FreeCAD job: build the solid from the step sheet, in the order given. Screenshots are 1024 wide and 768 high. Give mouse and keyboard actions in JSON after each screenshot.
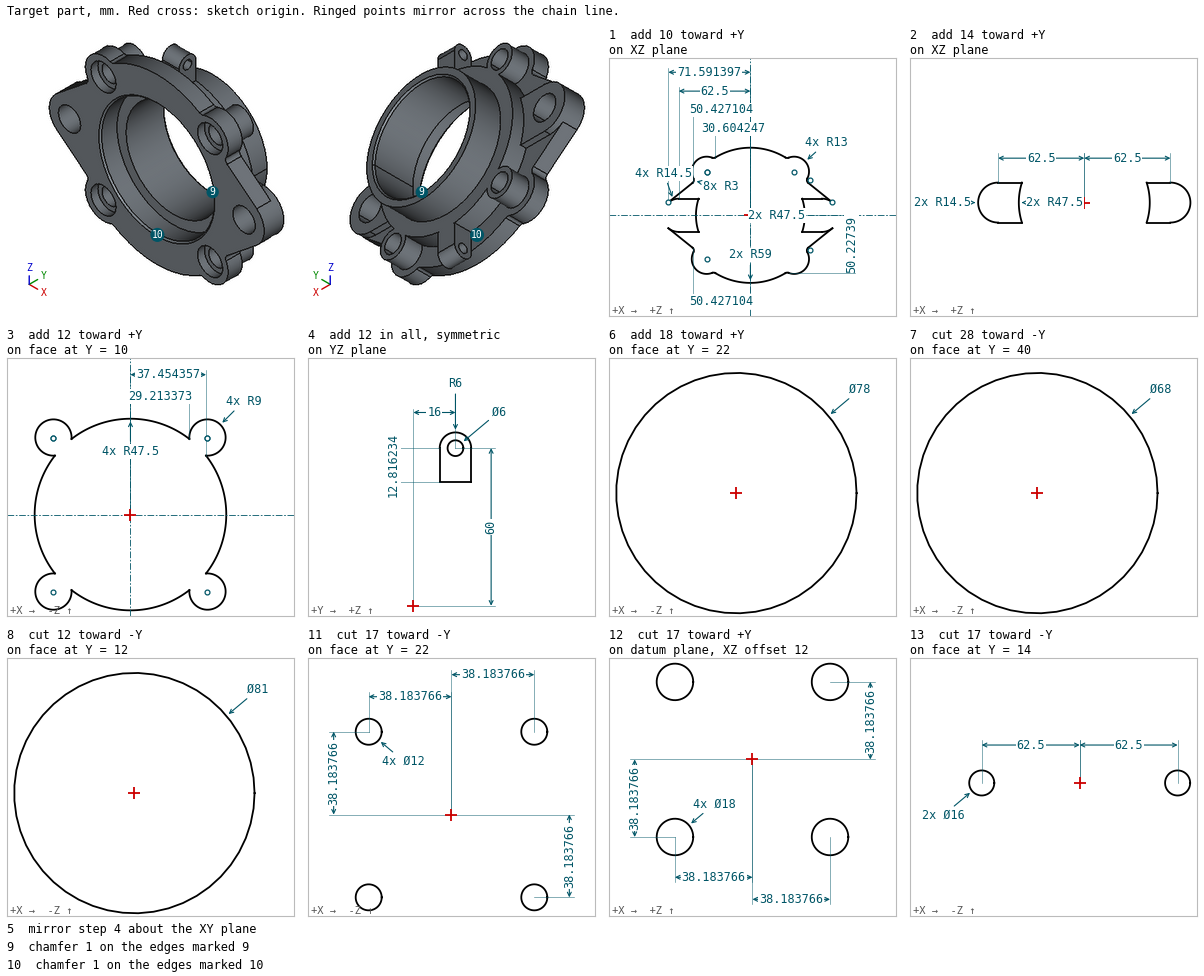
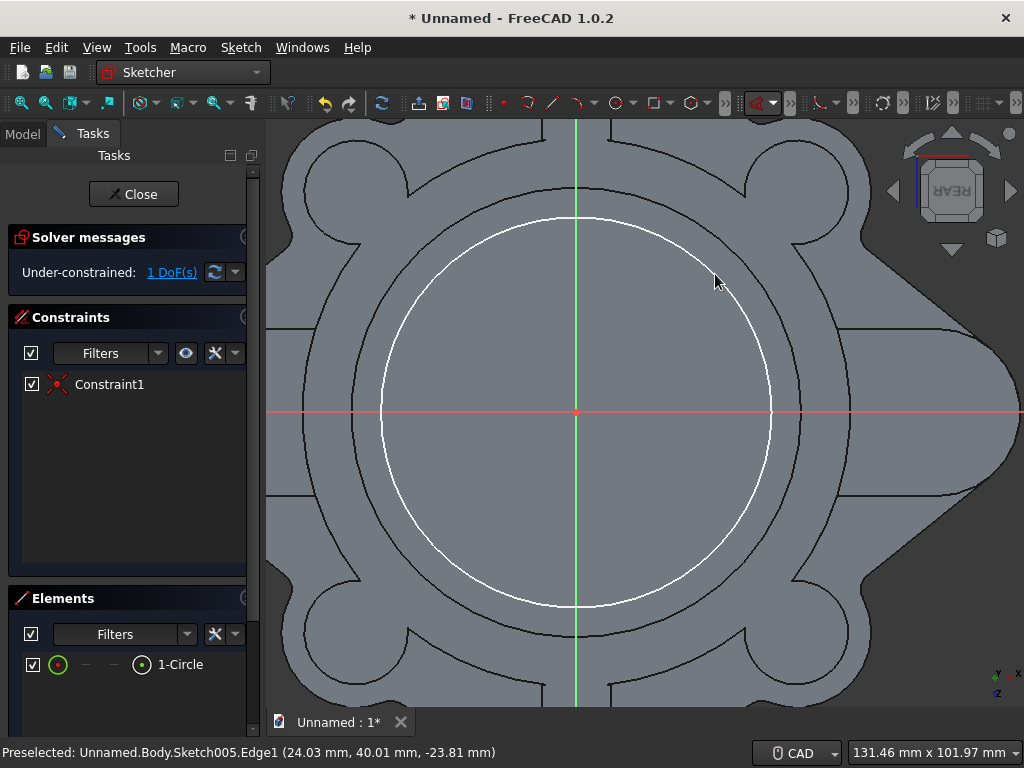
{"action": "key", "text": "d"}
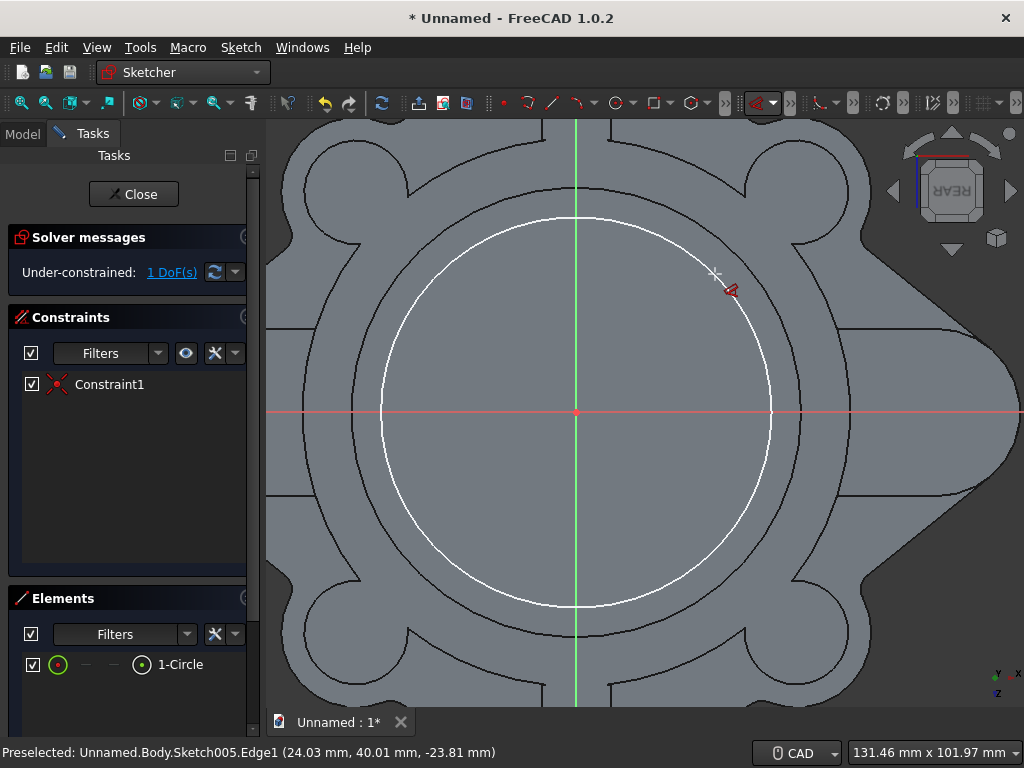
{"action": "left_click", "coordinate": [714, 274]}
{"action": "left_click", "coordinate": [737, 251]}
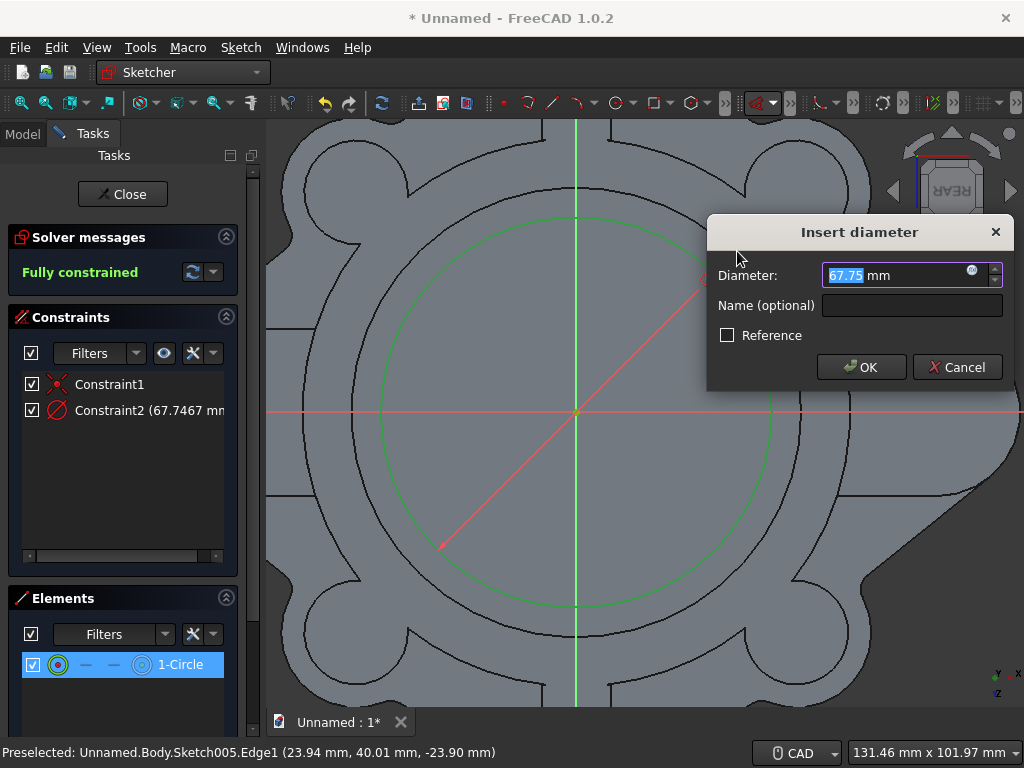
{"action": "type", "text": "68"}
{"action": "key", "text": "Return"}
{"action": "key", "text": "Escape"}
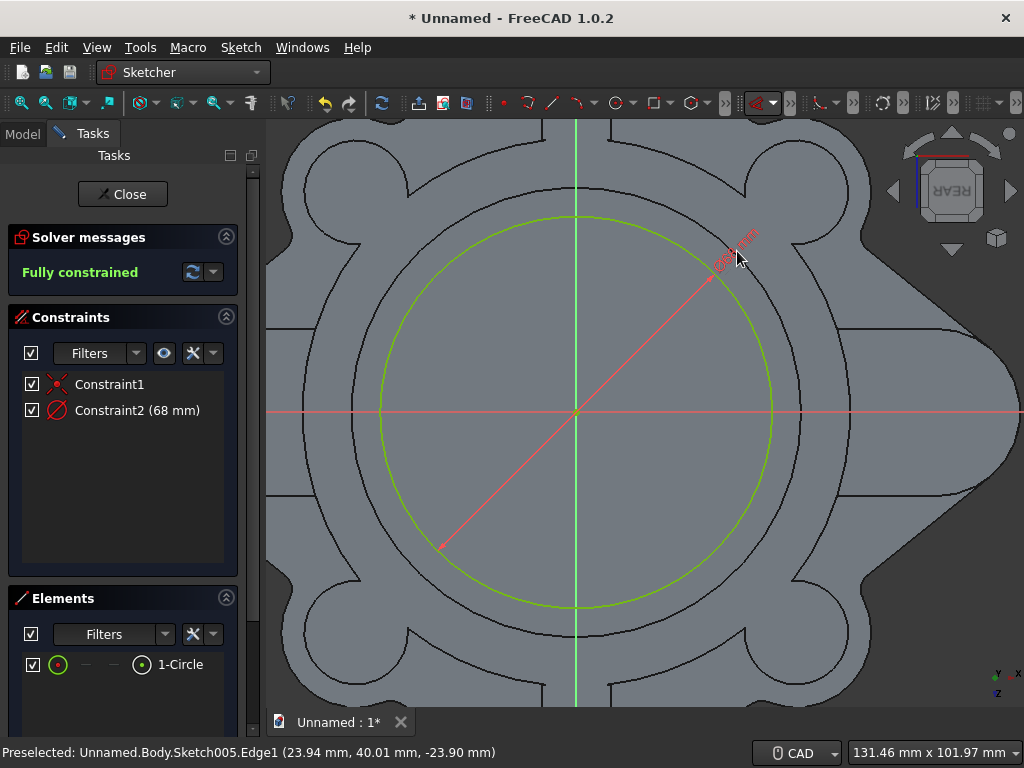
{"action": "left_click", "coordinate": [123, 194]}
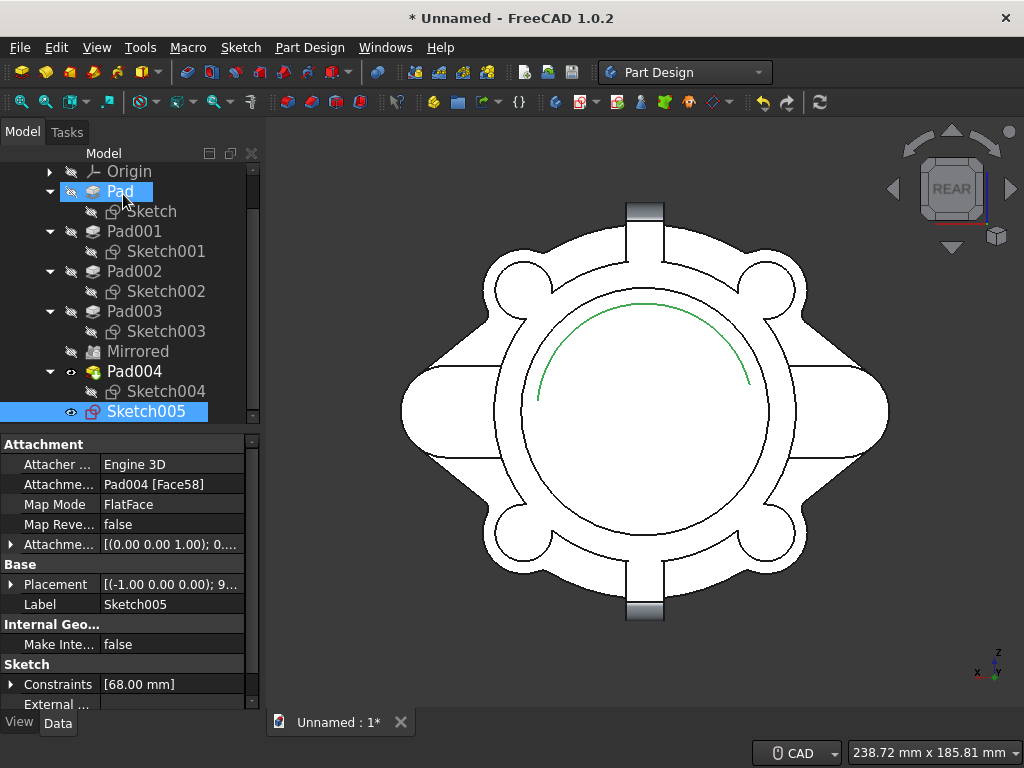
{"action": "left_click", "coordinate": [188, 72]}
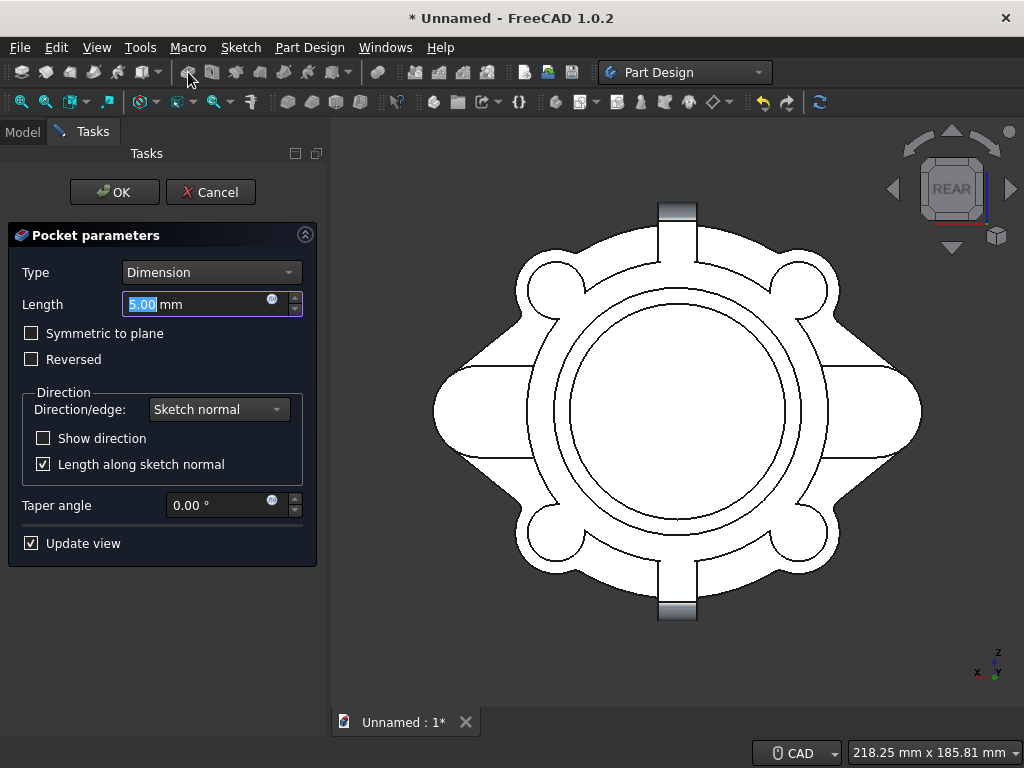
{"action": "type", "text": "28"}
{"action": "key", "text": "Tab"}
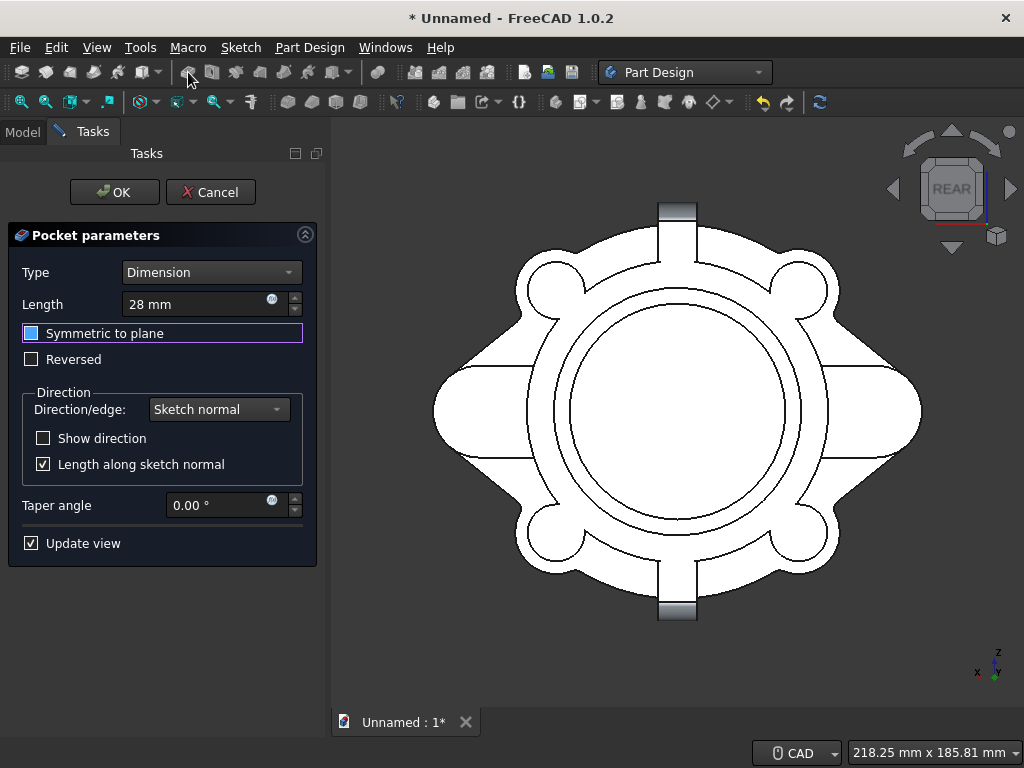
{"action": "left_click", "coordinate": [115, 192]}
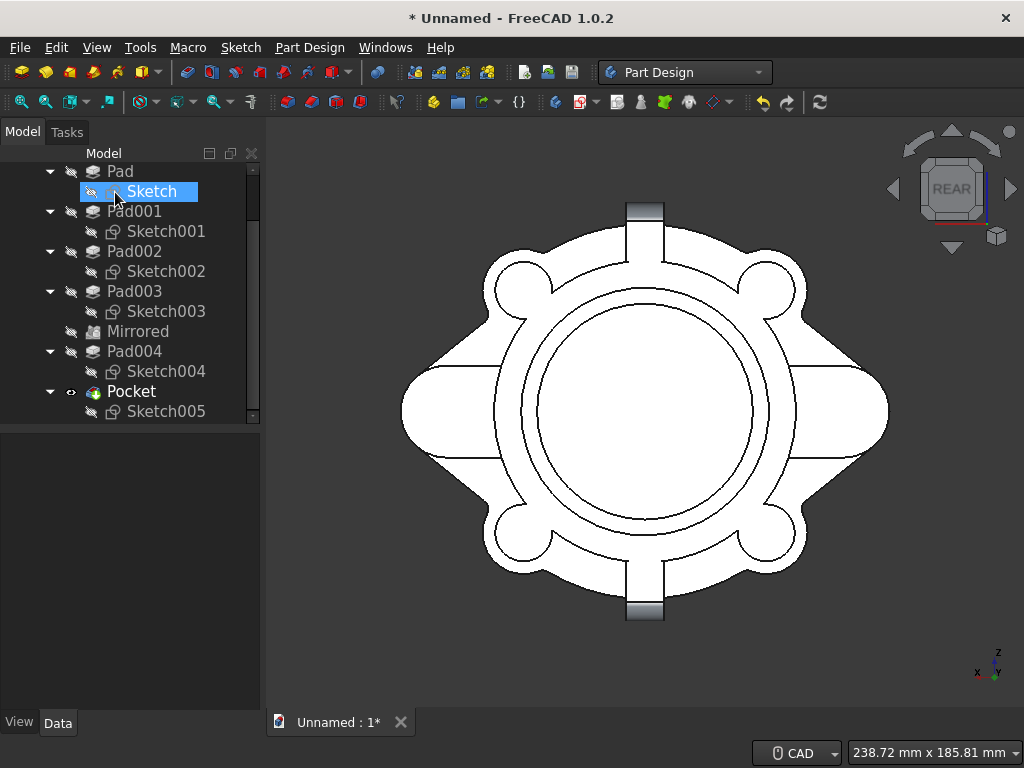
{"action": "left_click", "coordinate": [645, 411]}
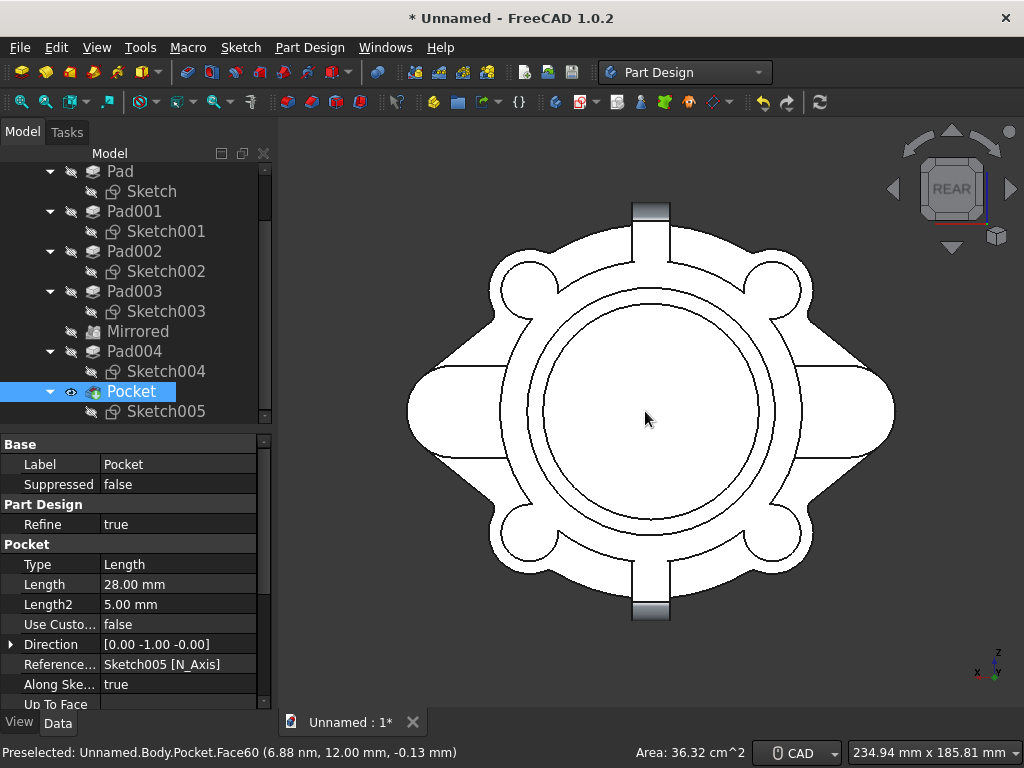
{"action": "left_click", "coordinate": [580, 102]}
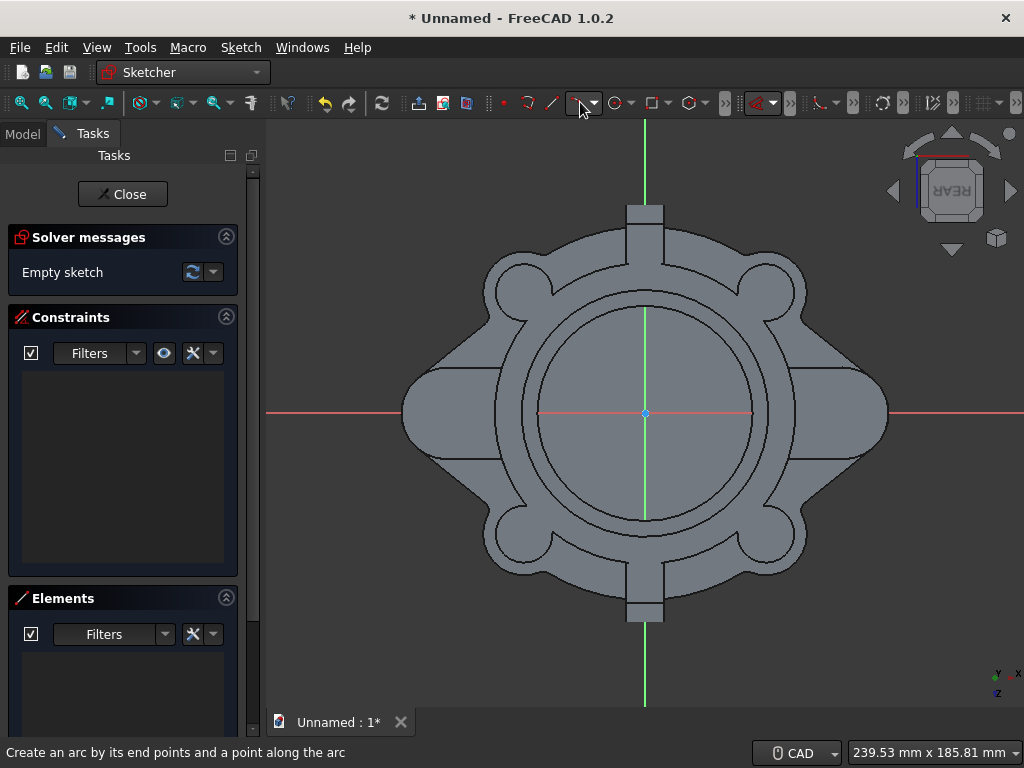
{"action": "scroll", "coordinate": [784, 414], "scroll_direction": "up", "scroll_amount": 2}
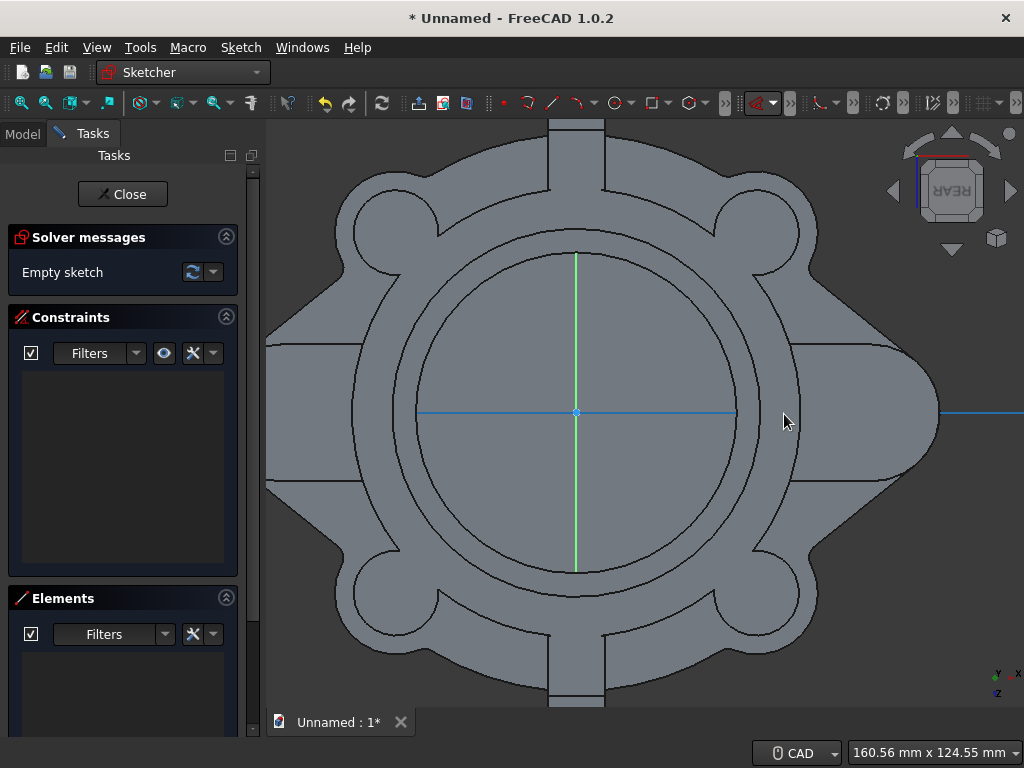
{"action": "key", "text": "g c"}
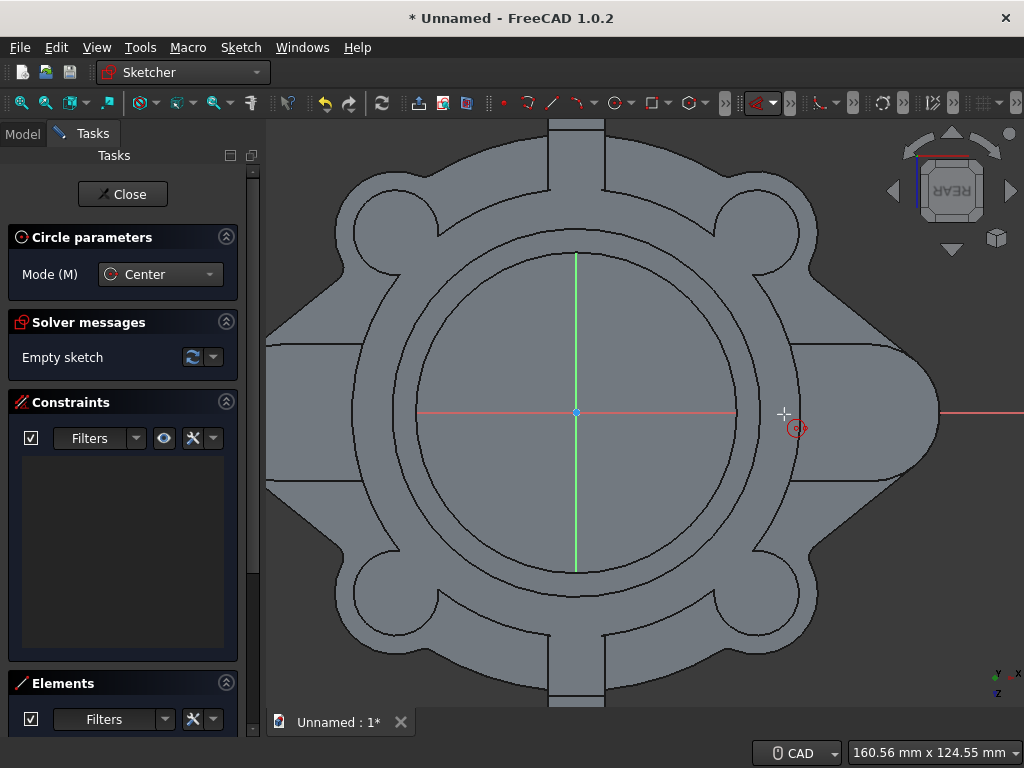
{"action": "left_click", "coordinate": [576, 413]}
{"action": "left_click", "coordinate": [711, 278]}
{"action": "key", "text": "Escape"}